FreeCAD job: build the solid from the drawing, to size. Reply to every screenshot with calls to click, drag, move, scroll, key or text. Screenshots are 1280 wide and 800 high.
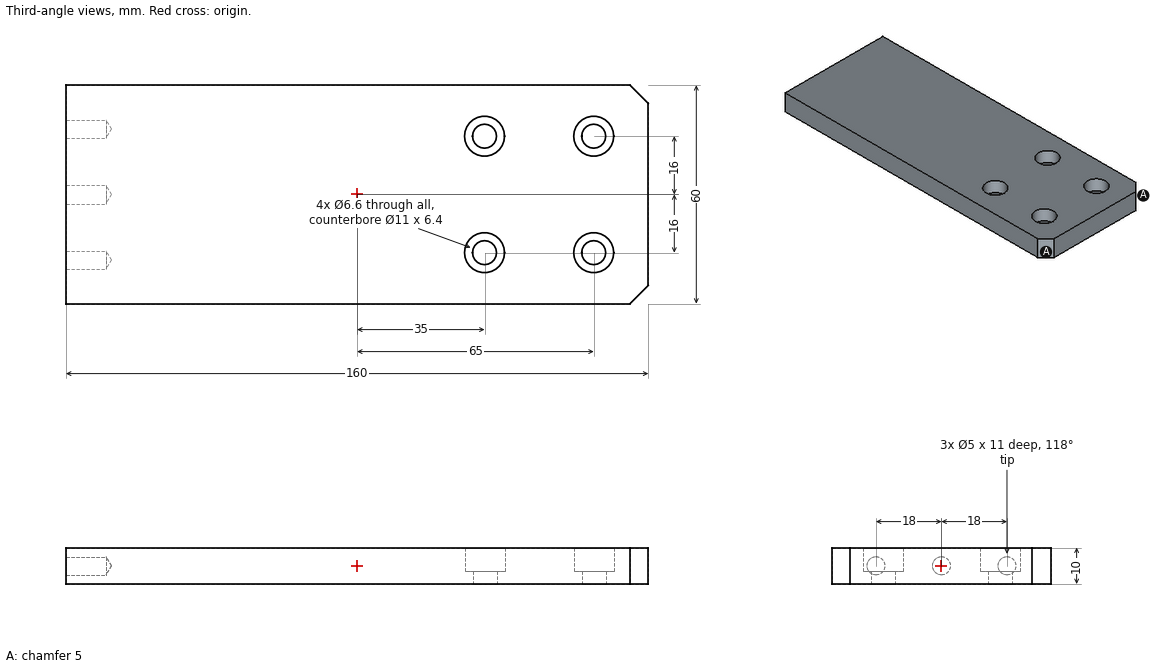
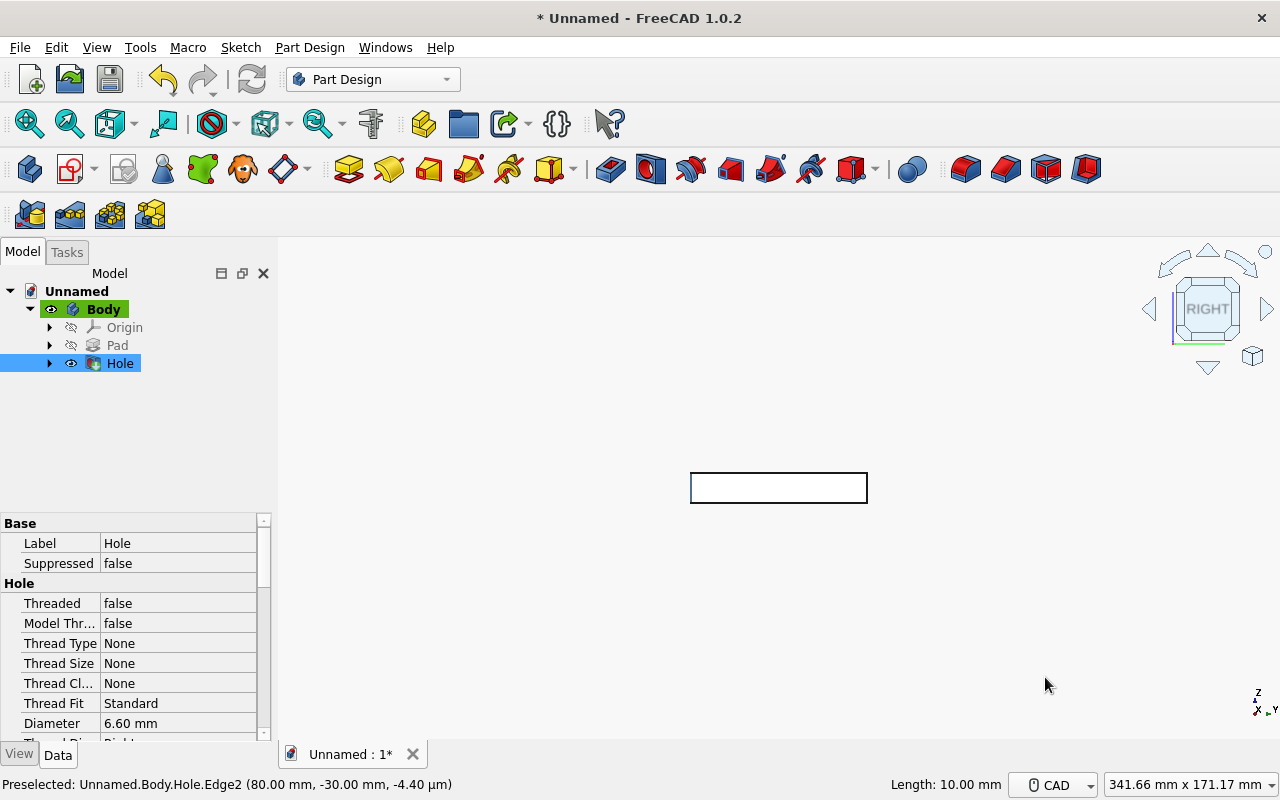
click(867, 487, ctrl)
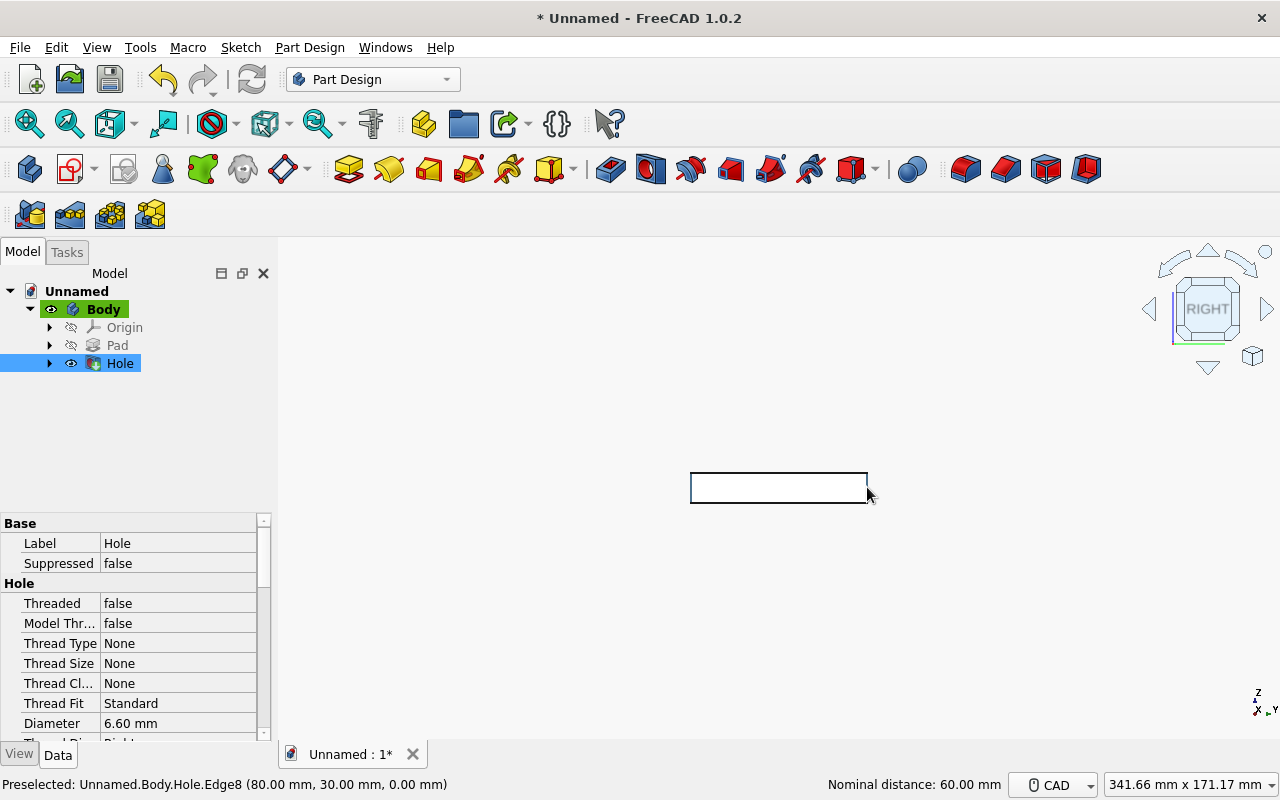
click(1006, 170)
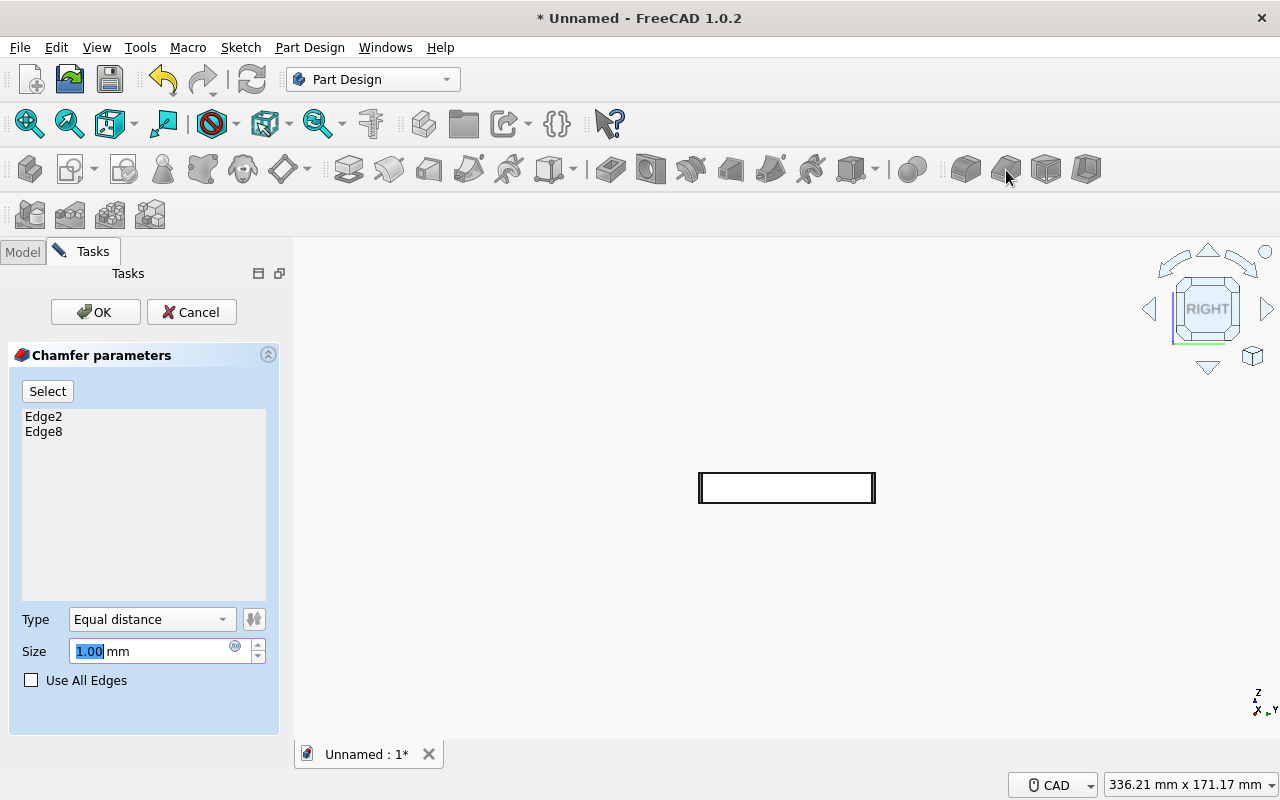
text(5)
key(Tab)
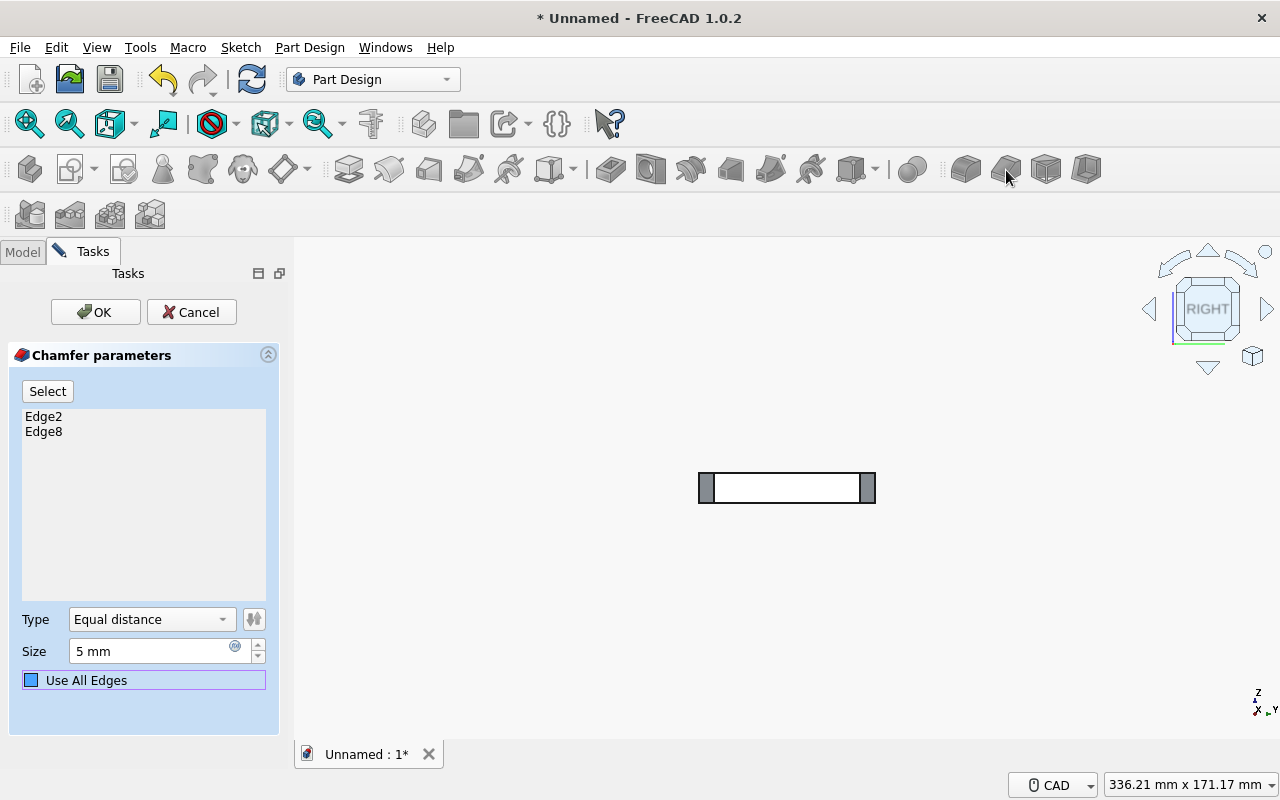
click(96, 312)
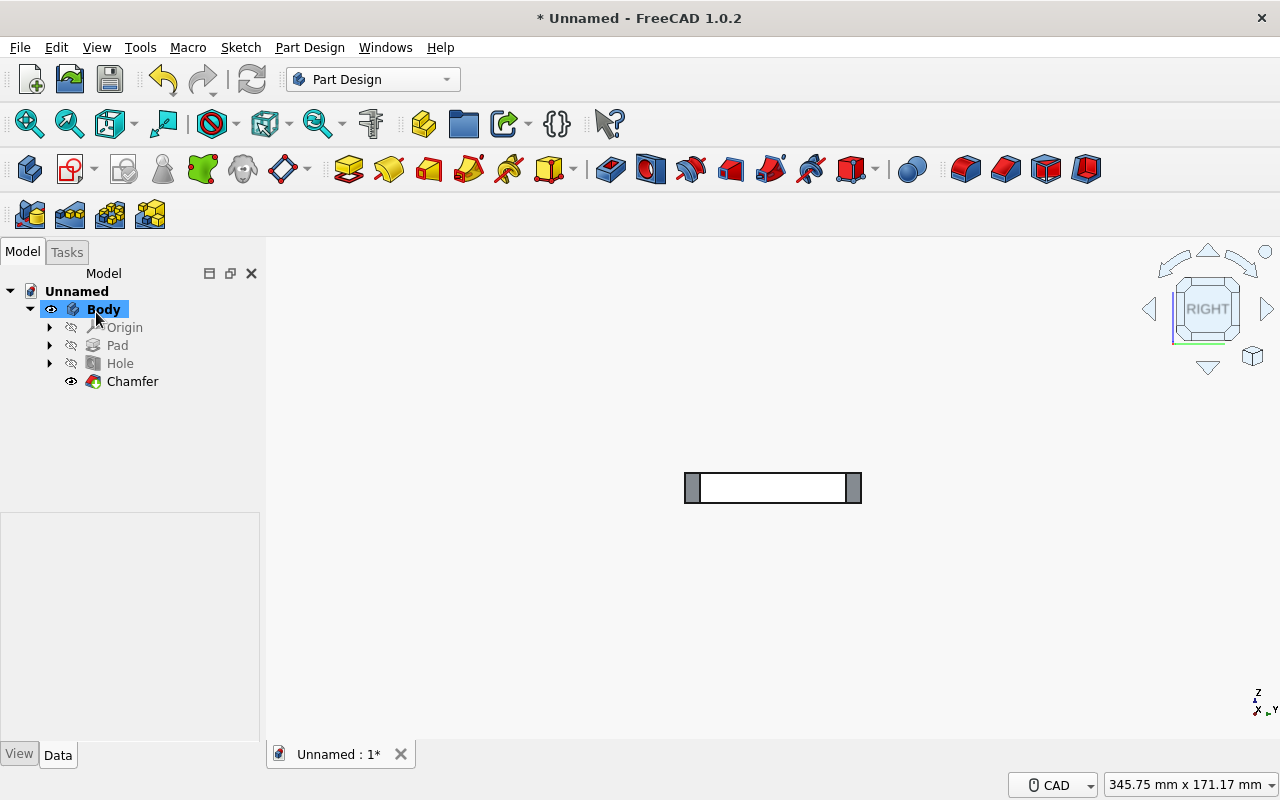
key(v)
key(f)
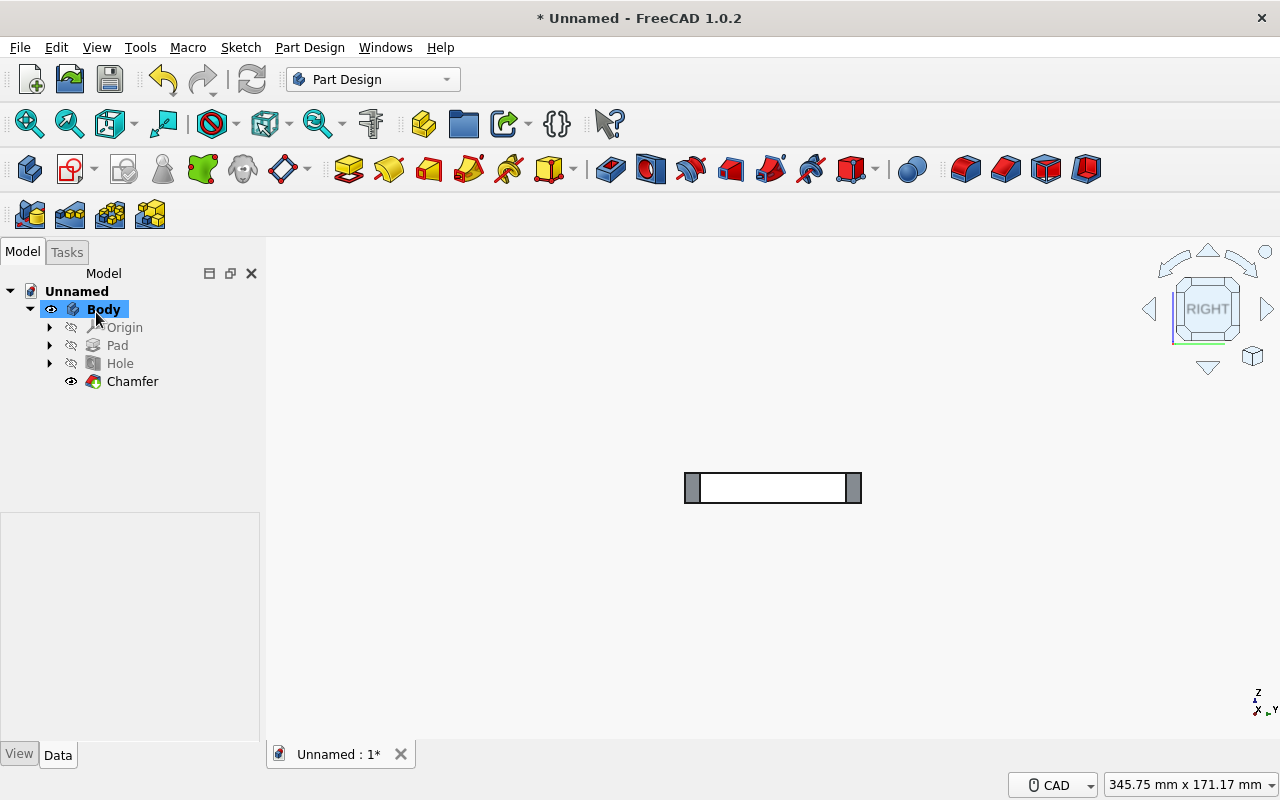
key(6)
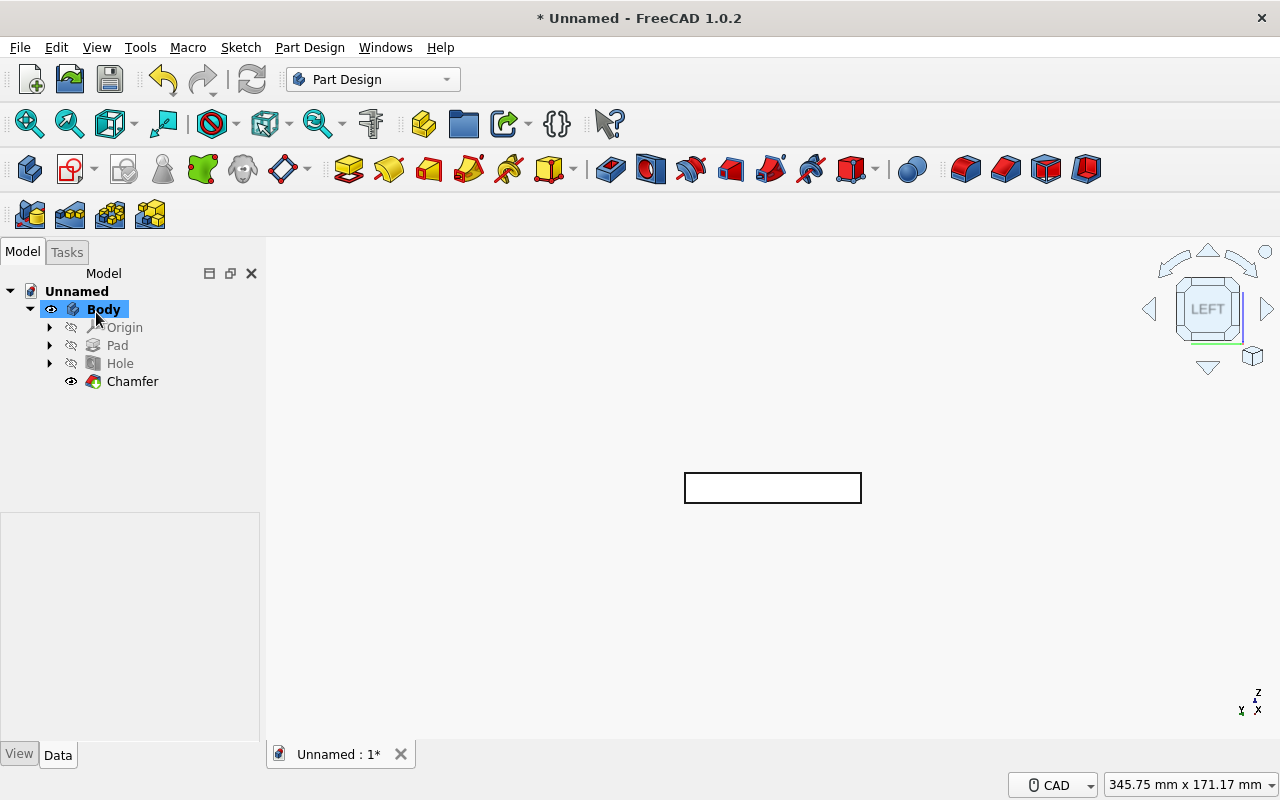
click(30, 124)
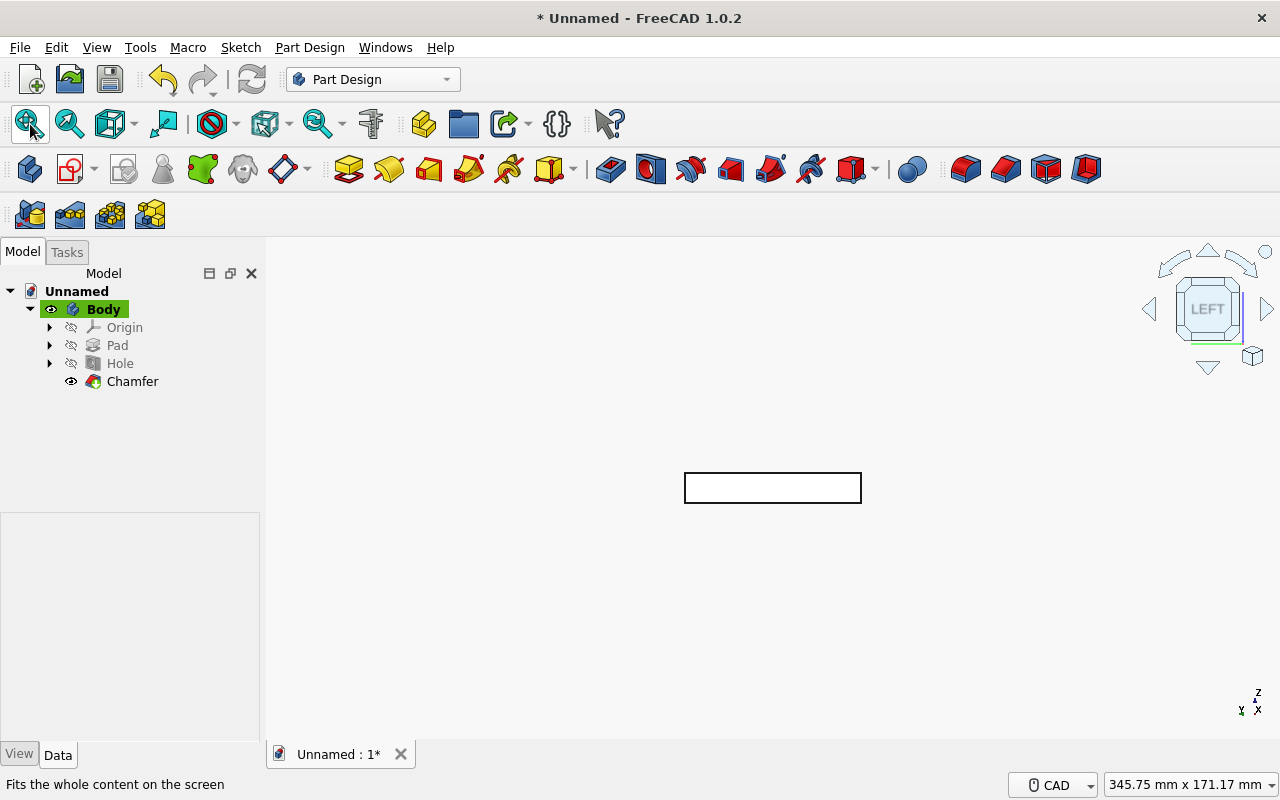
click(723, 487)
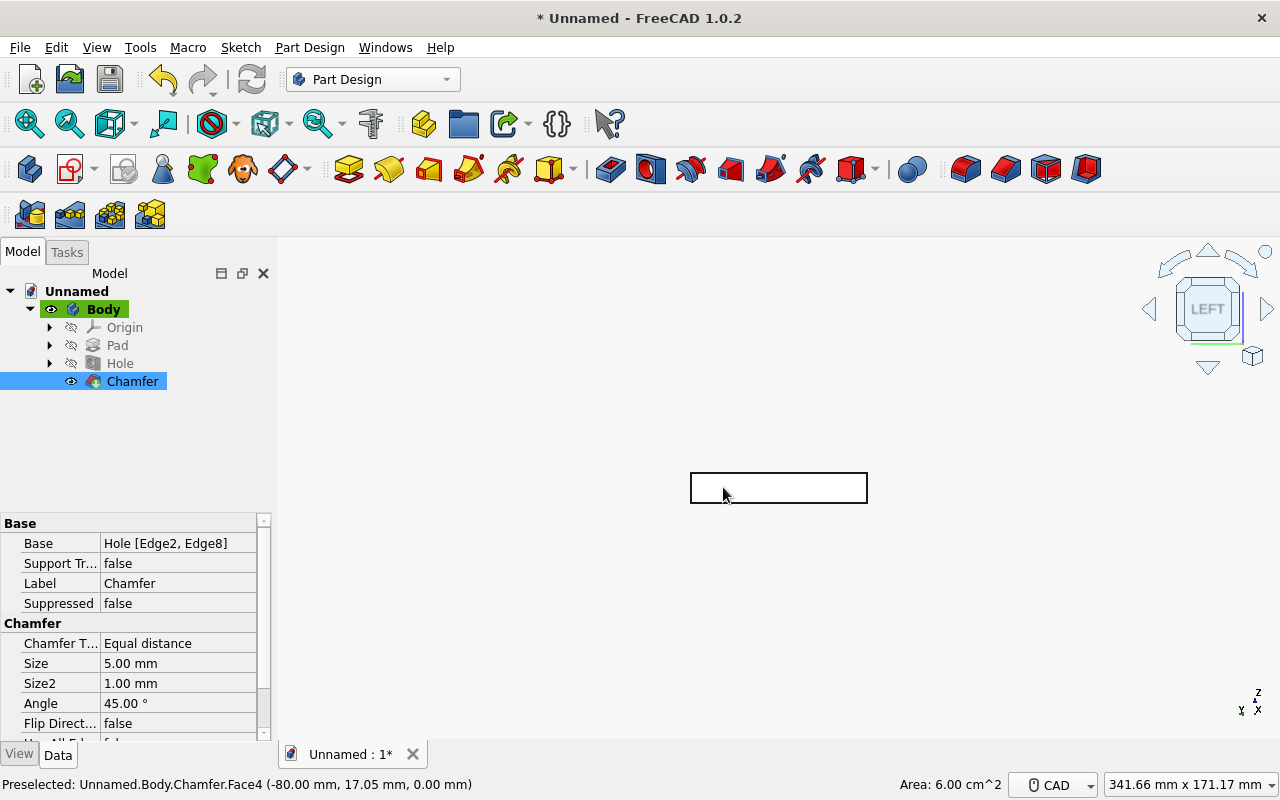
click(70, 170)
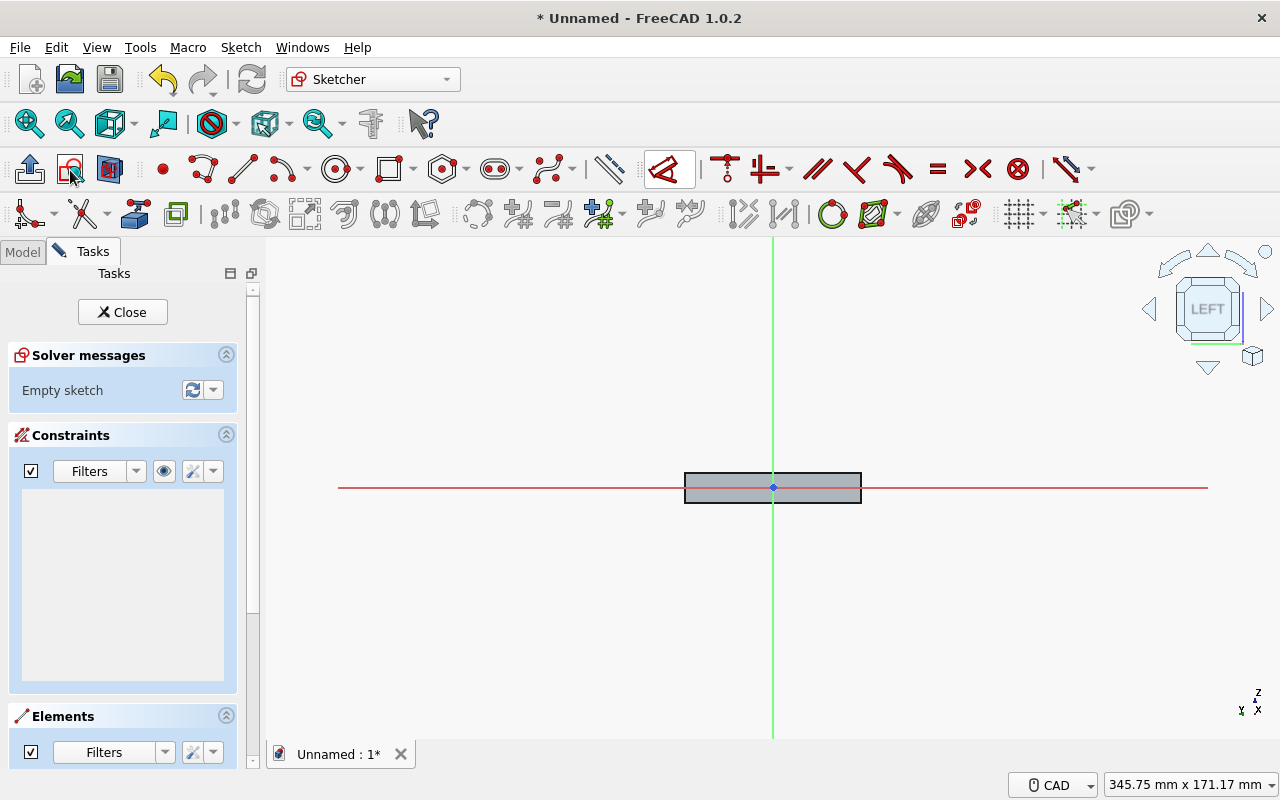
scroll(790, 488, up, 8)